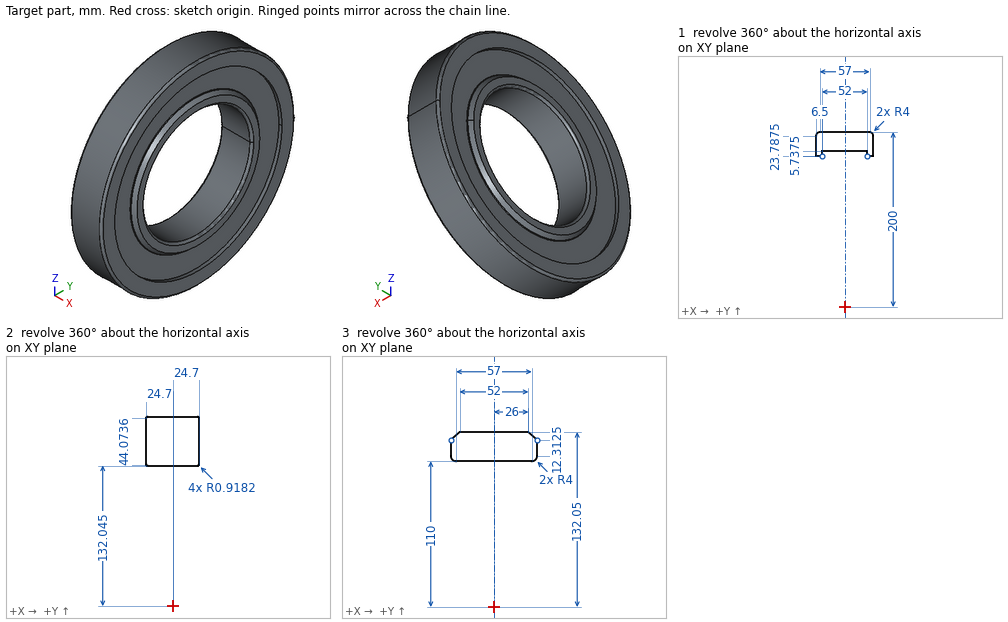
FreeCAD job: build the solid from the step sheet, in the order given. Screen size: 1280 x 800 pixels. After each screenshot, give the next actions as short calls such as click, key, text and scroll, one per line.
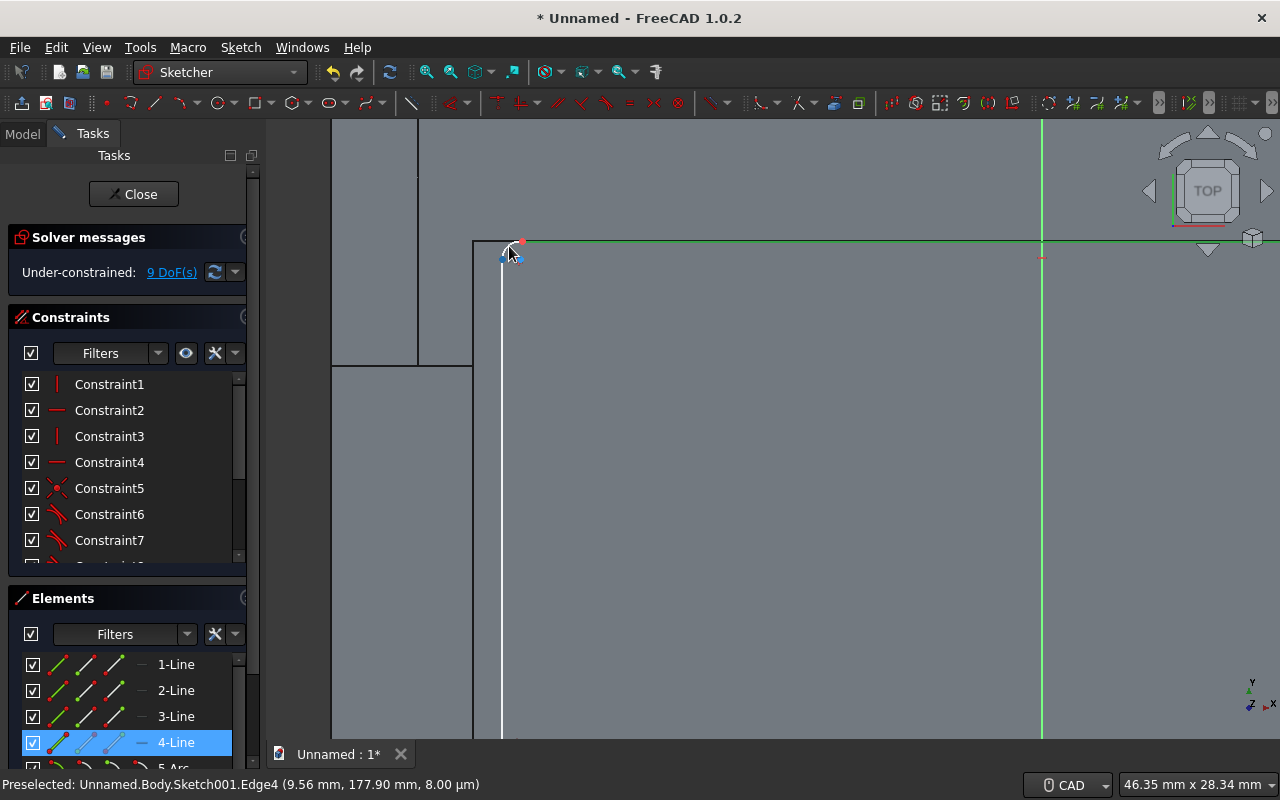
click(508, 246)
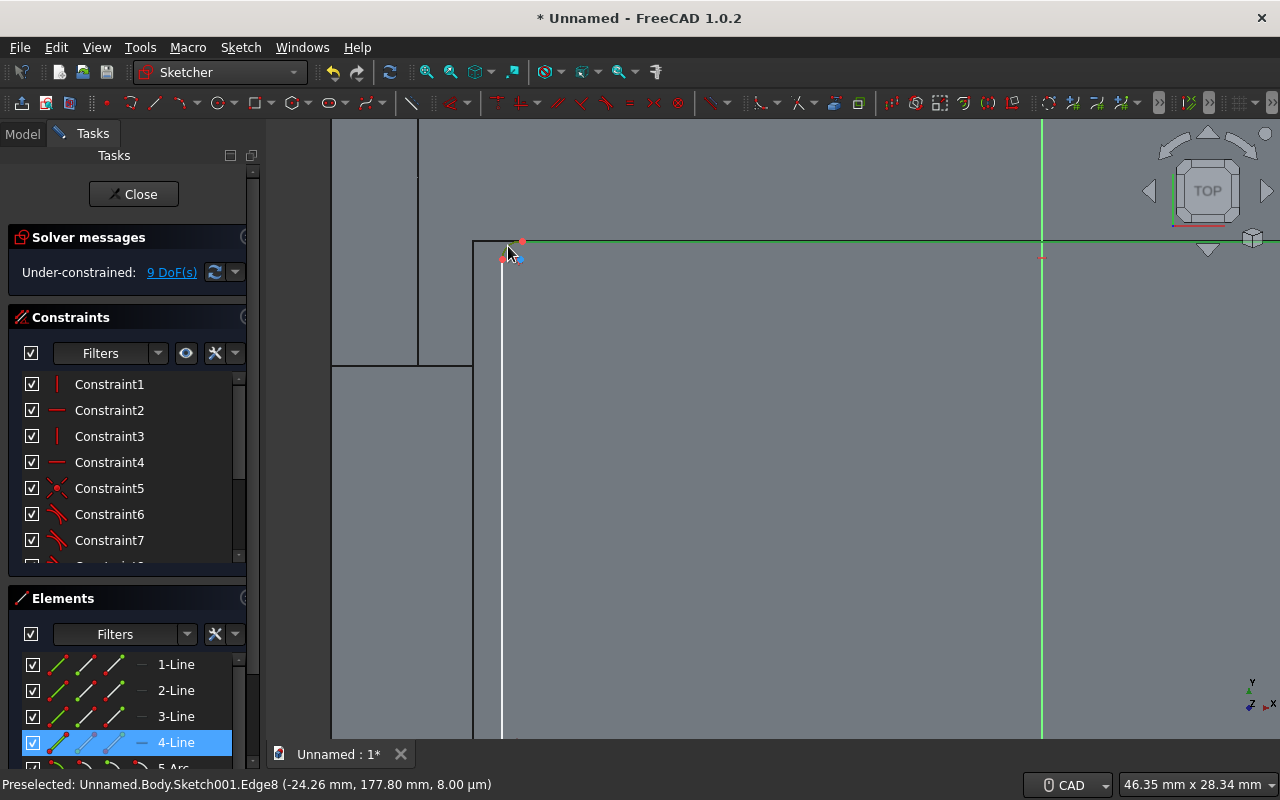
click(606, 104)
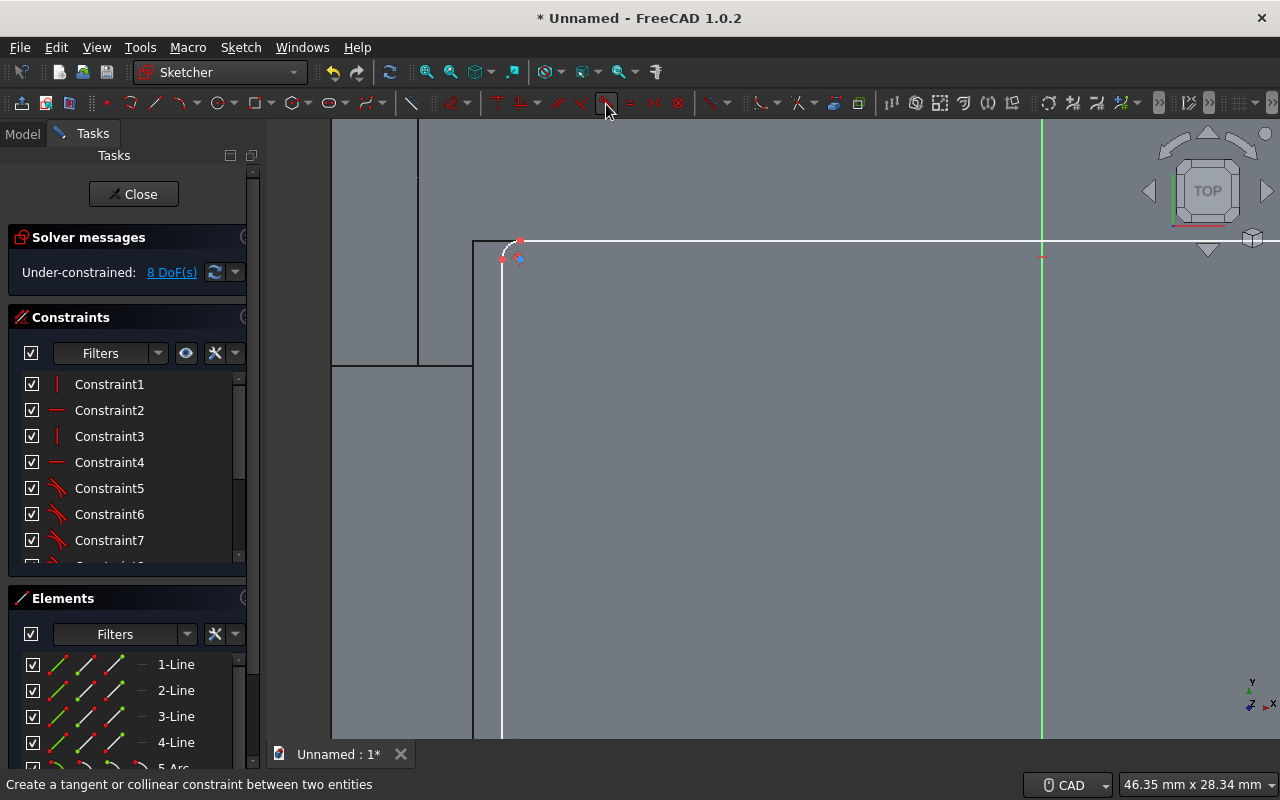
scroll(508, 246, down, 5)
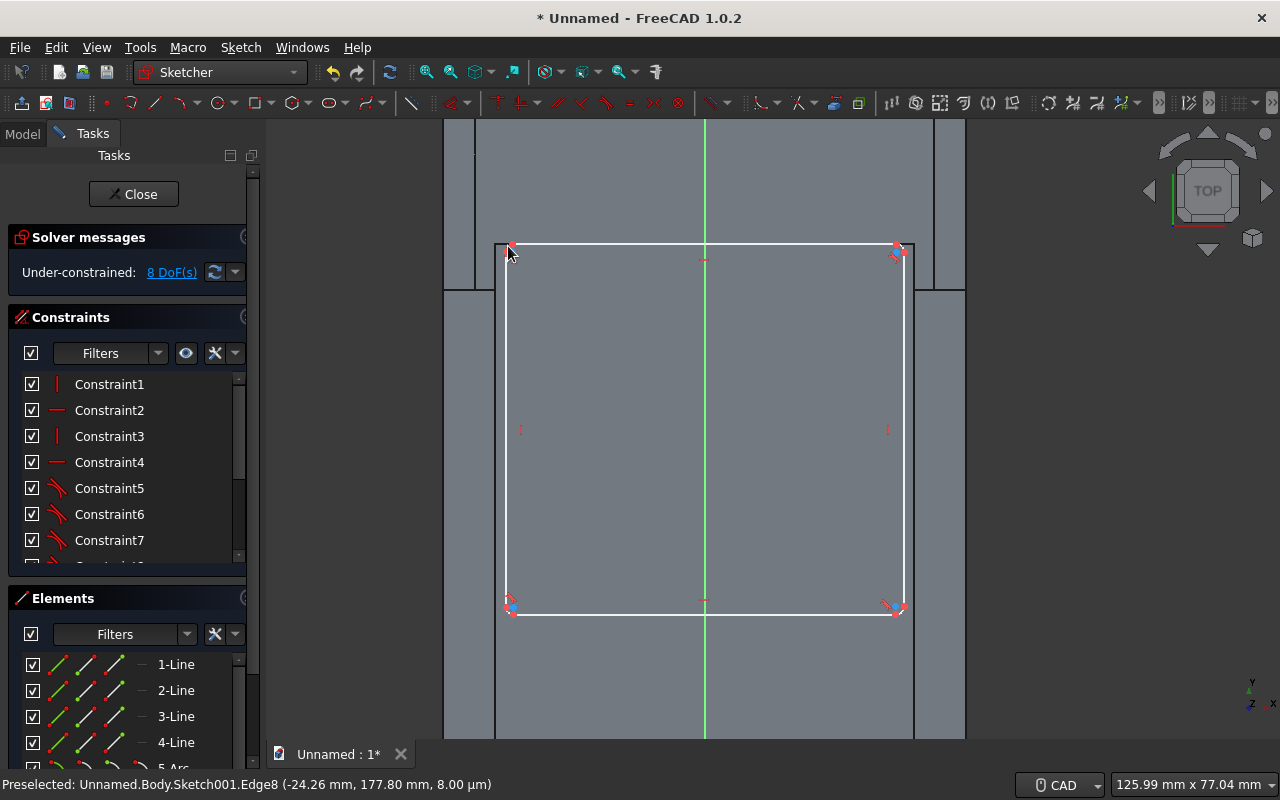
scroll(507, 611, up, 7)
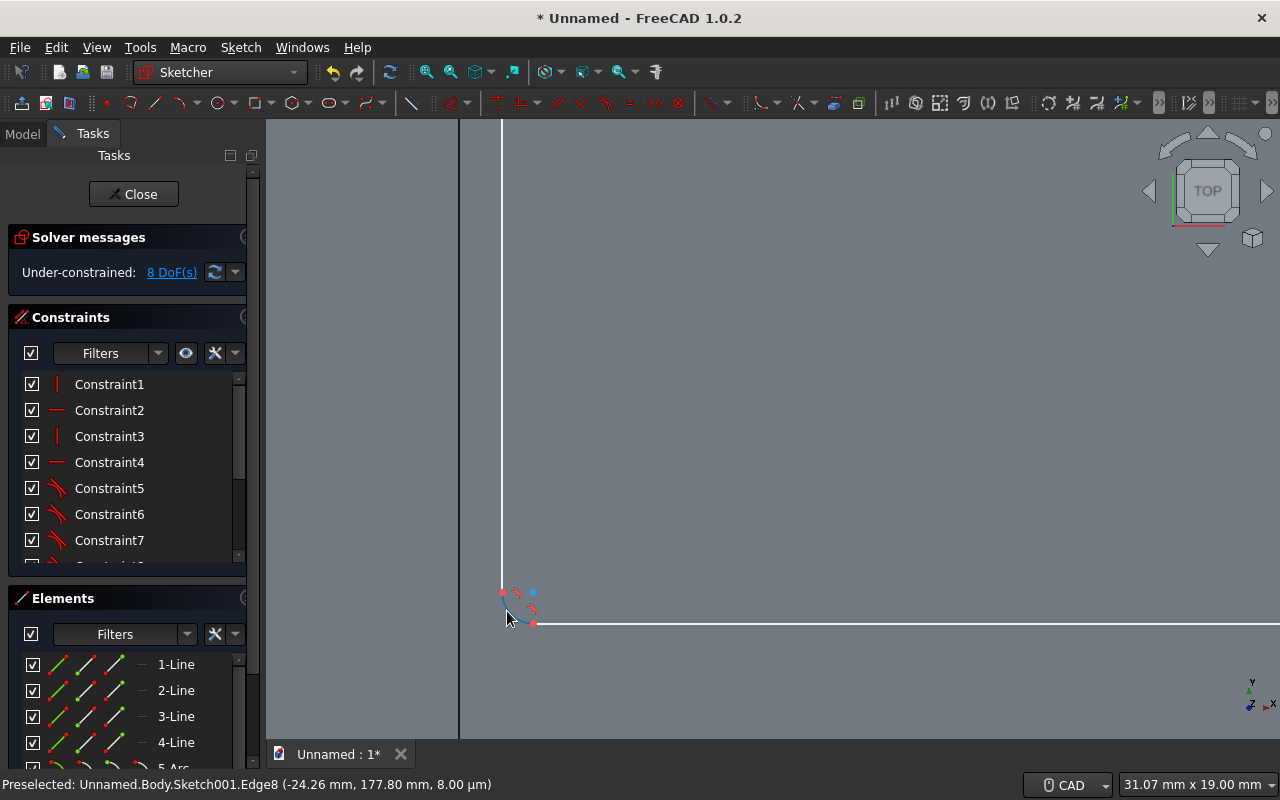
click(506, 607)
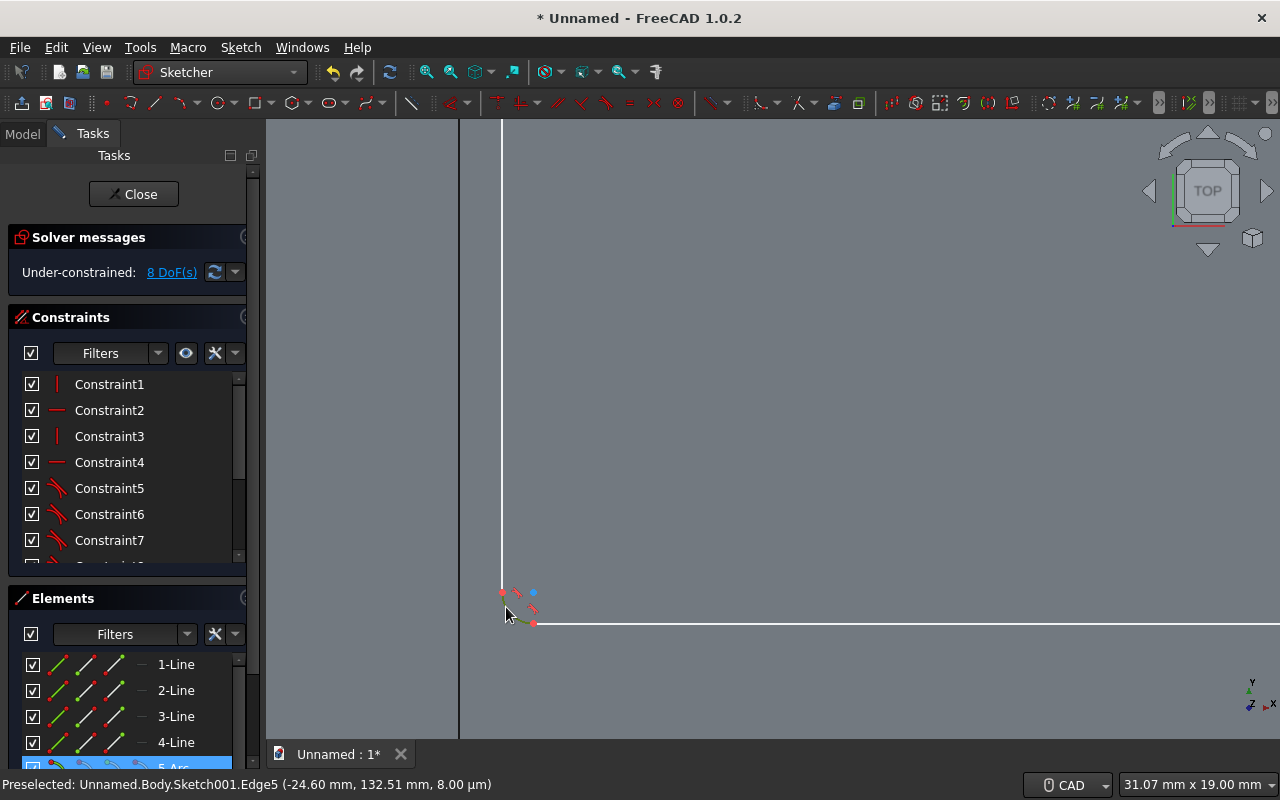
scroll(507, 612, down, 7)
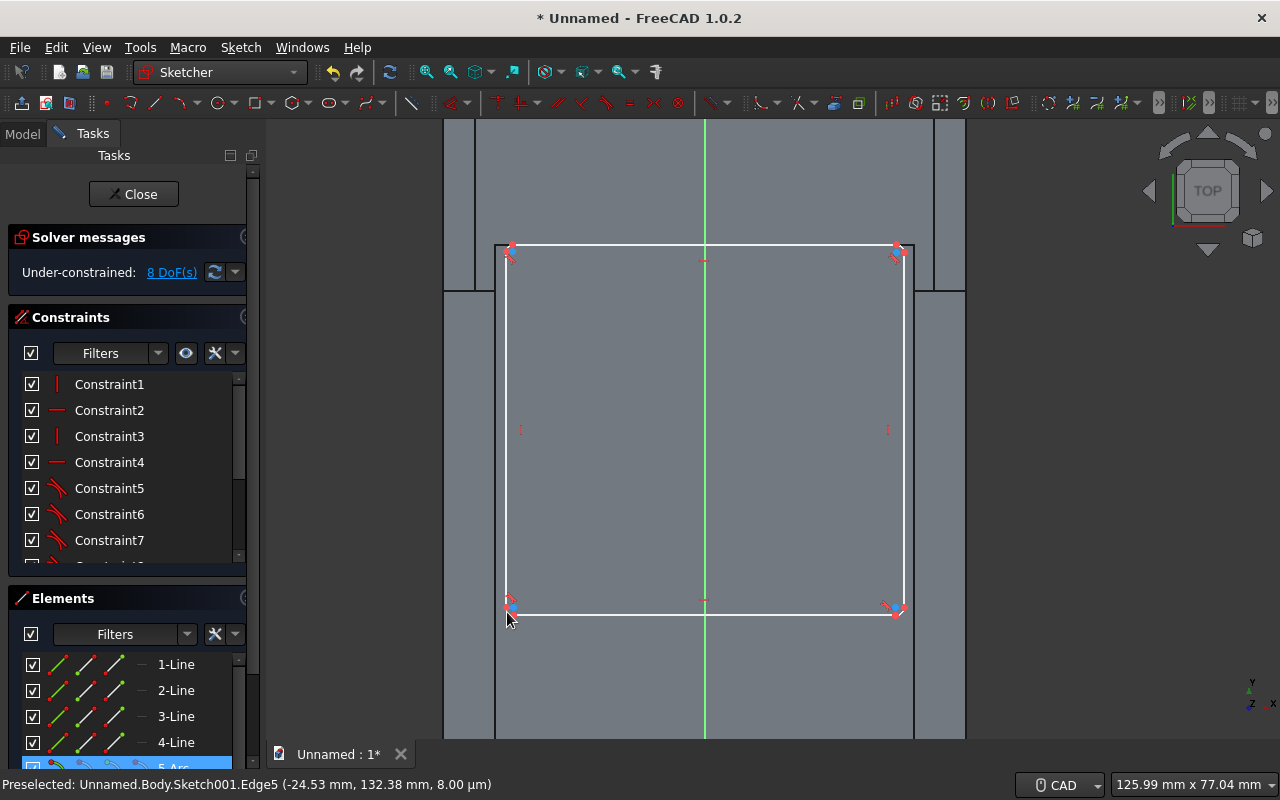
scroll(900, 615, up, 7)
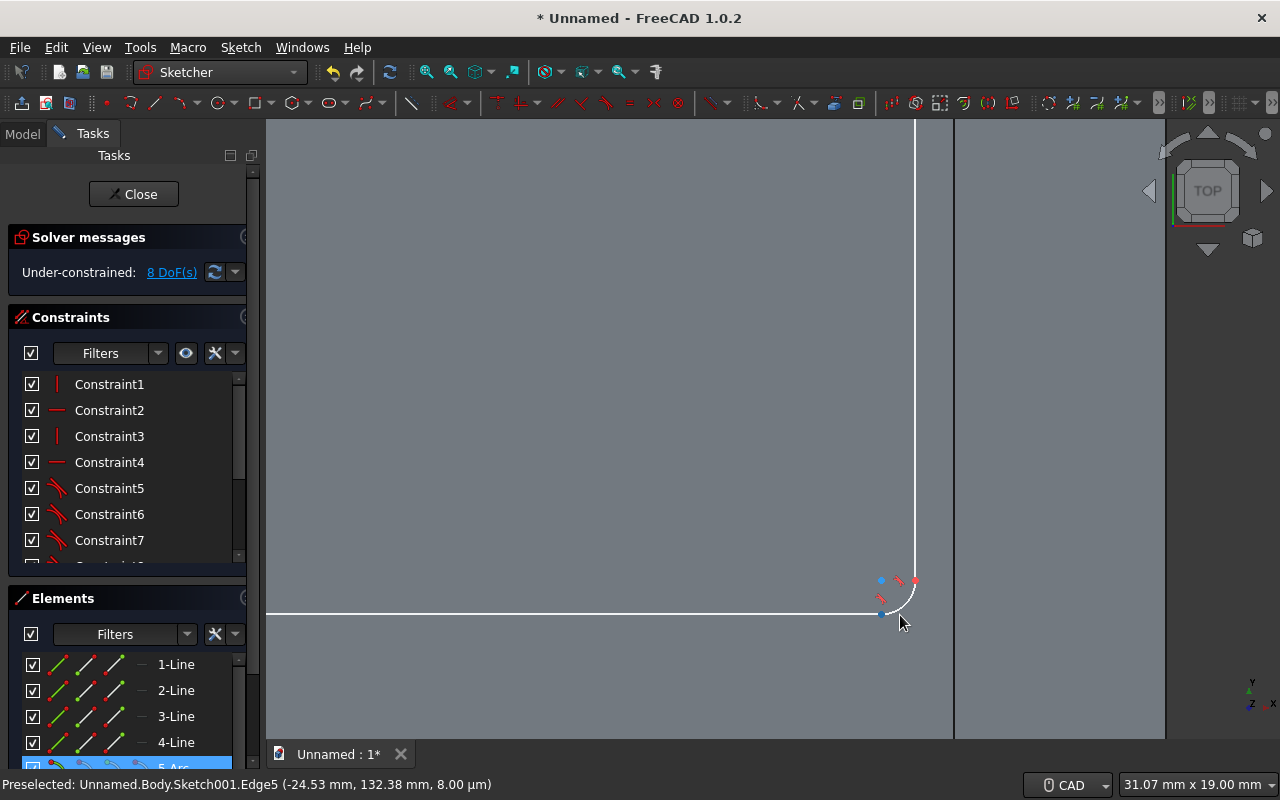
click(897, 611)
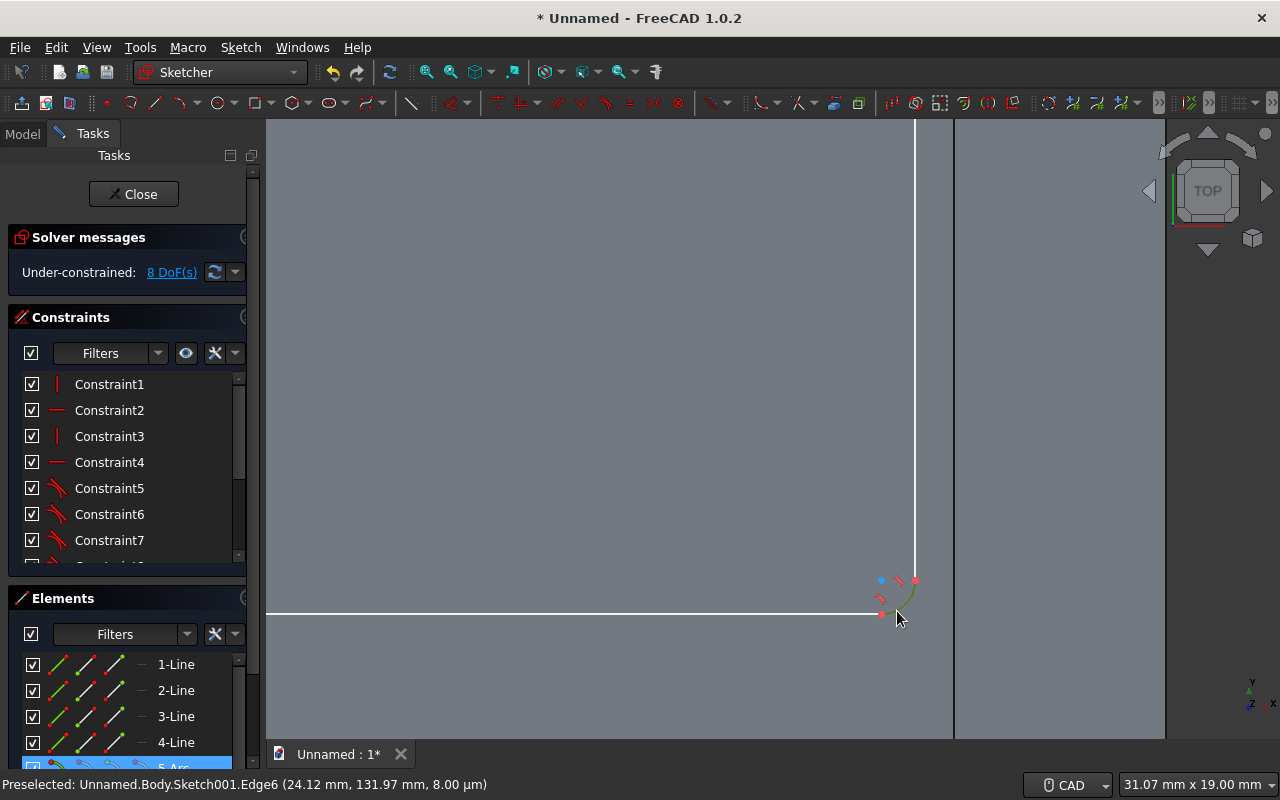
scroll(901, 615, down, 7)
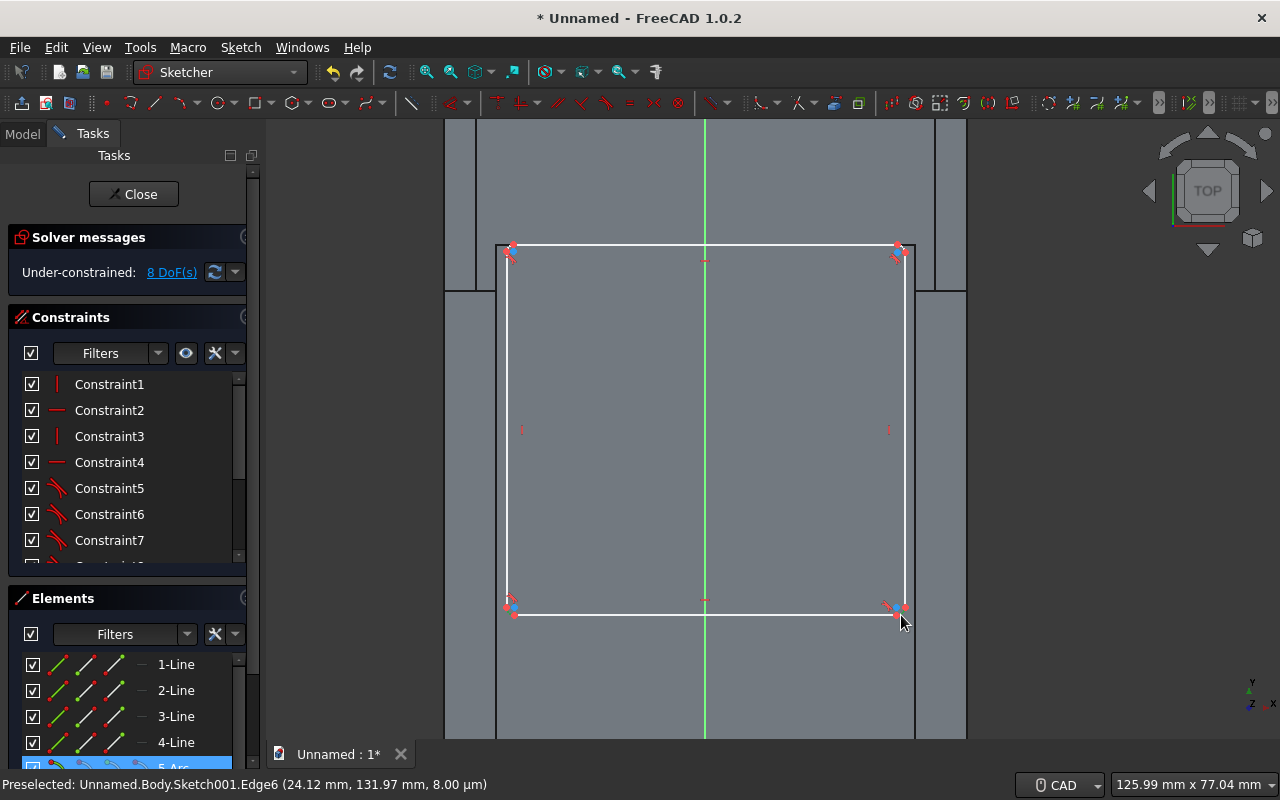
scroll(904, 249, up, 7)